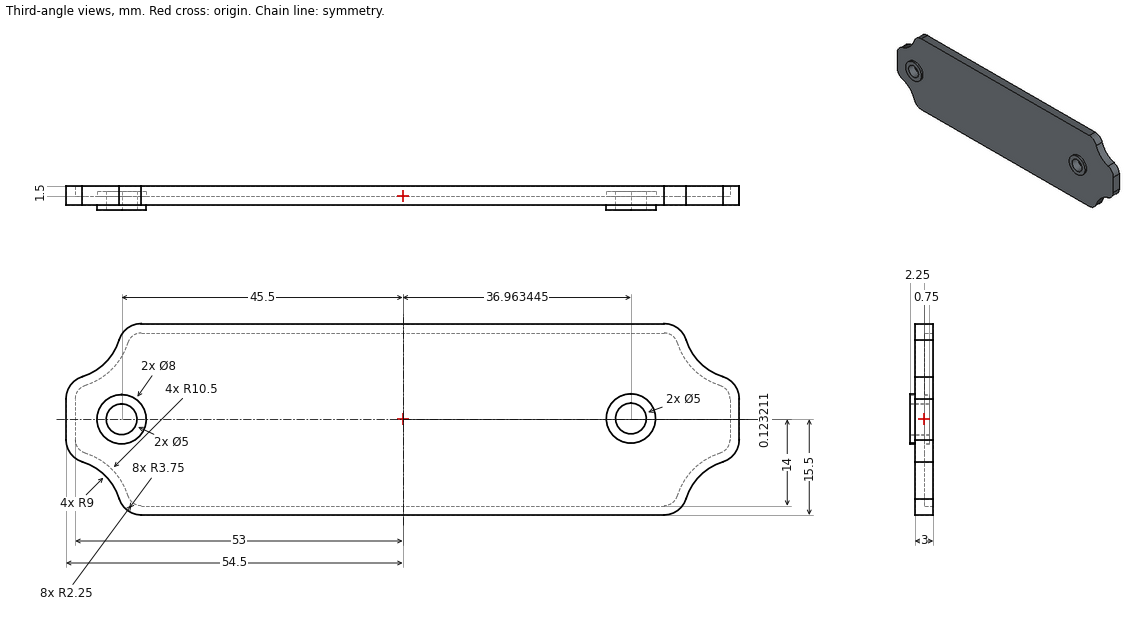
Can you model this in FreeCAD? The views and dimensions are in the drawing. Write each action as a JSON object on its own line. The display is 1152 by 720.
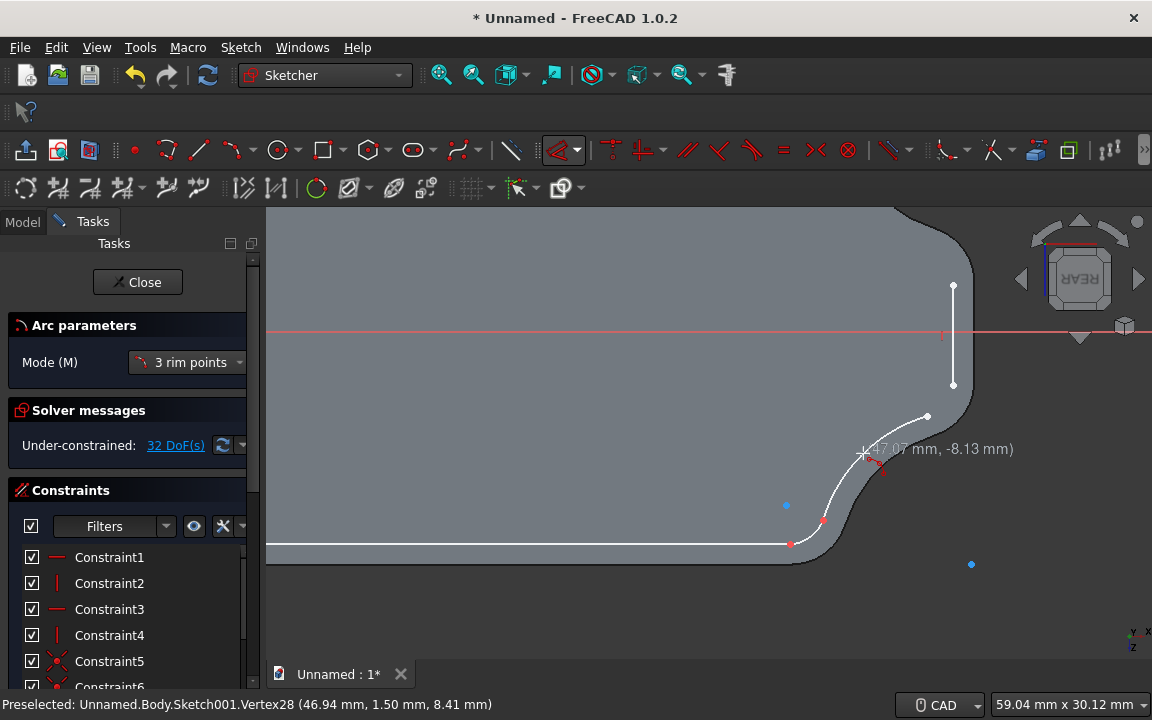
{"action": "left_click", "coordinate": [927, 416]}
{"action": "left_click", "coordinate": [953, 385]}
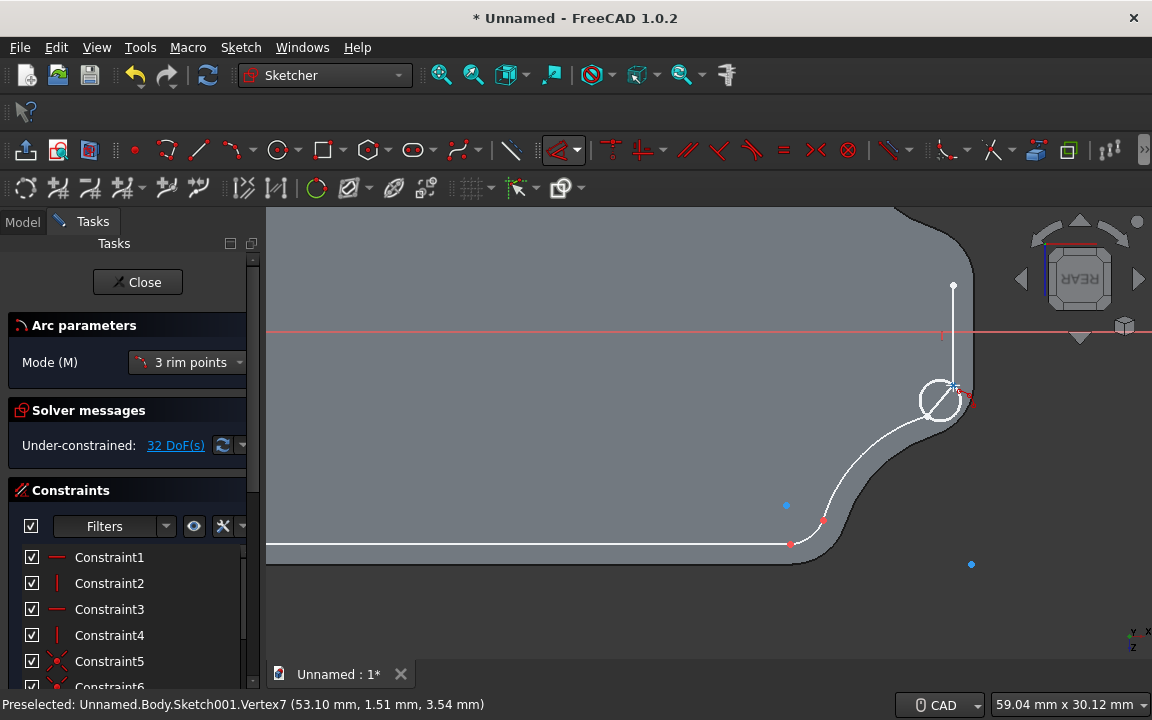
{"action": "scroll", "coordinate": [945, 402], "scroll_direction": "up", "scroll_amount": 5}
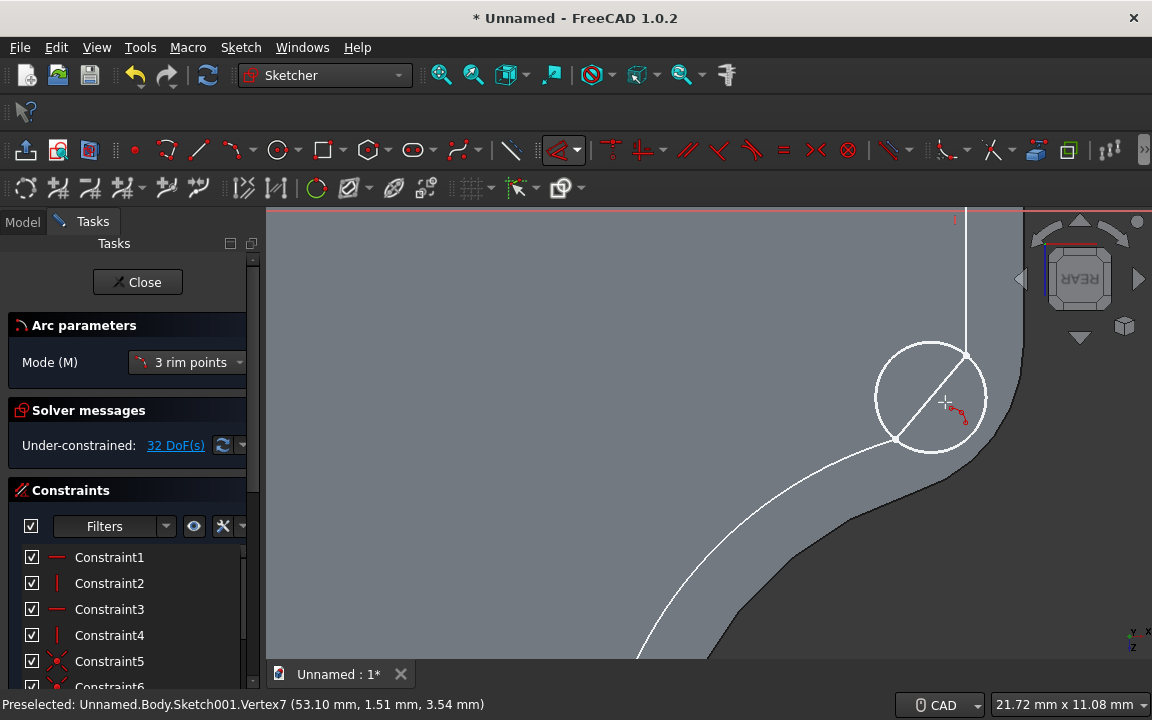
{"action": "left_click", "coordinate": [945, 401]}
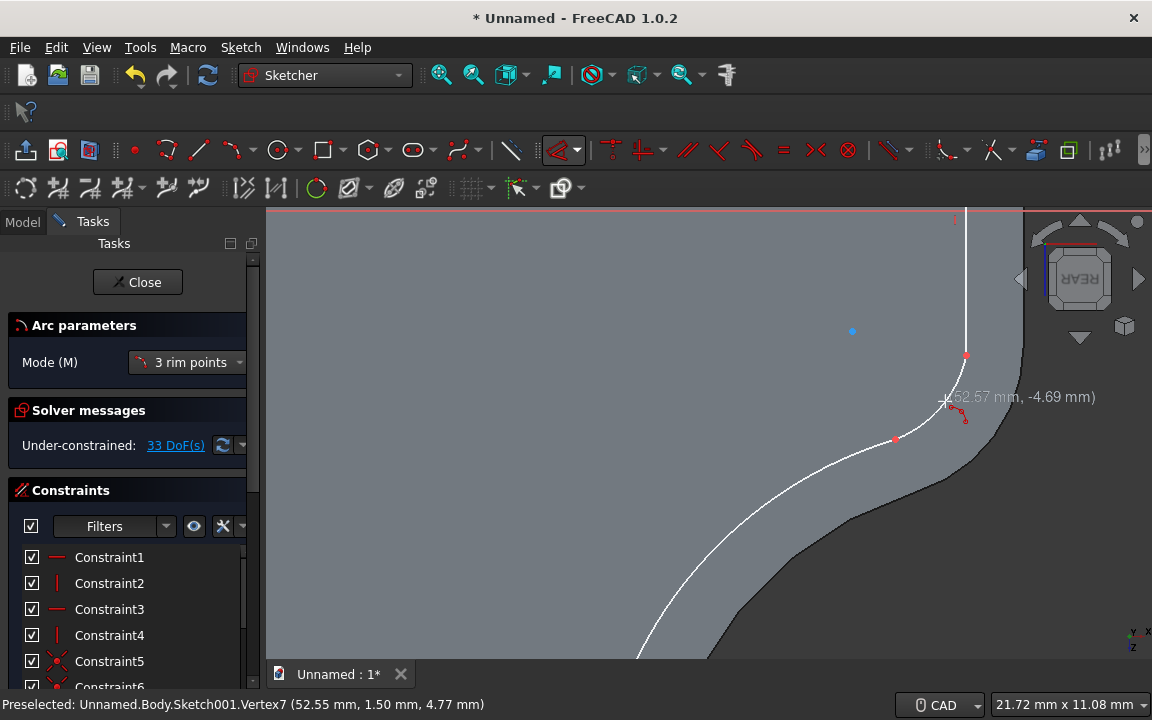
{"action": "scroll", "coordinate": [870, 461], "scroll_direction": "down", "scroll_amount": 11}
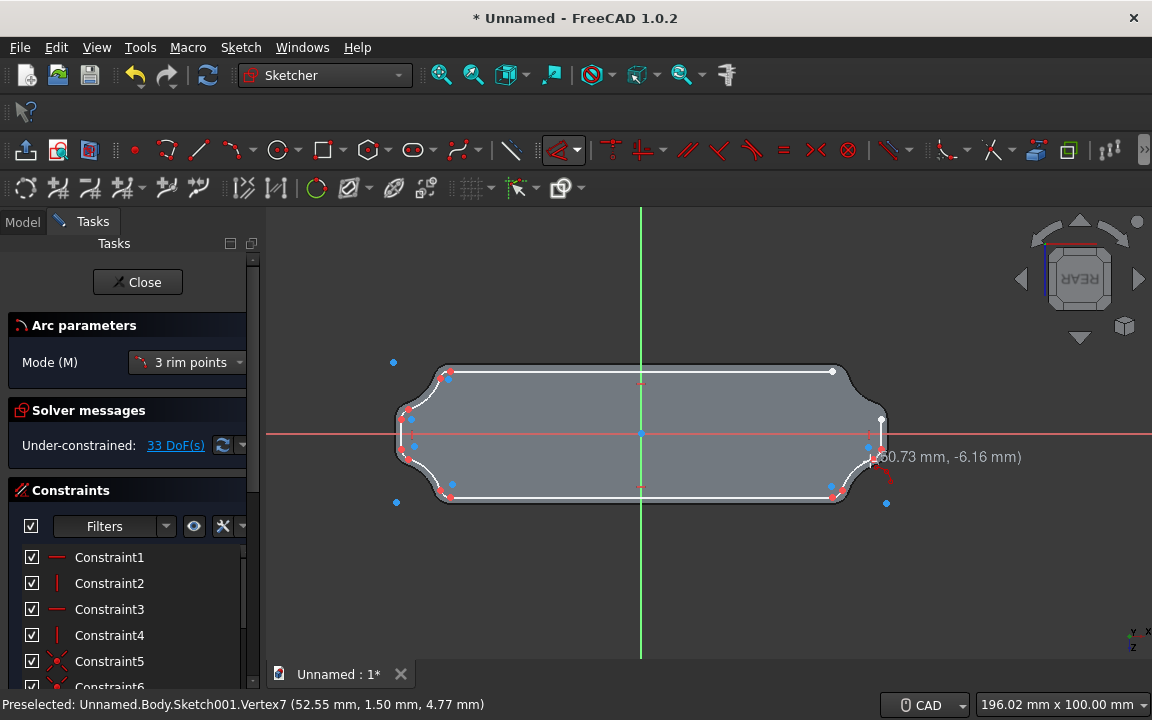
{"action": "left_click", "coordinate": [881, 420]}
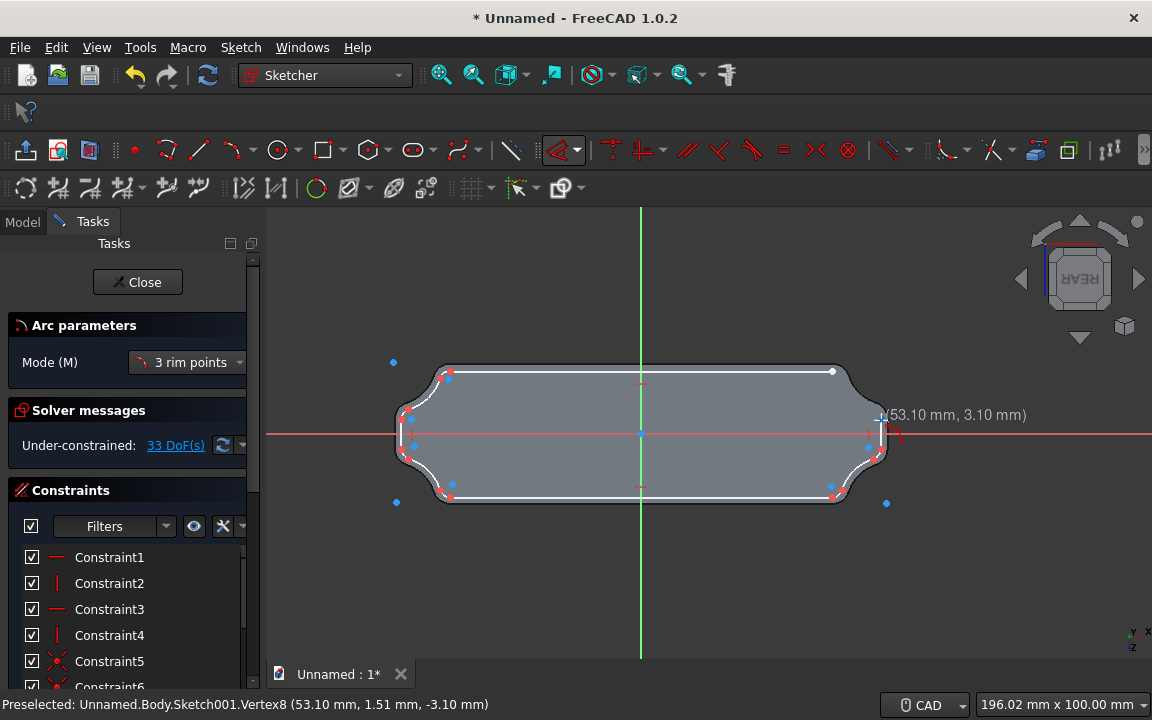
{"action": "scroll", "coordinate": [874, 409], "scroll_direction": "up", "scroll_amount": 2}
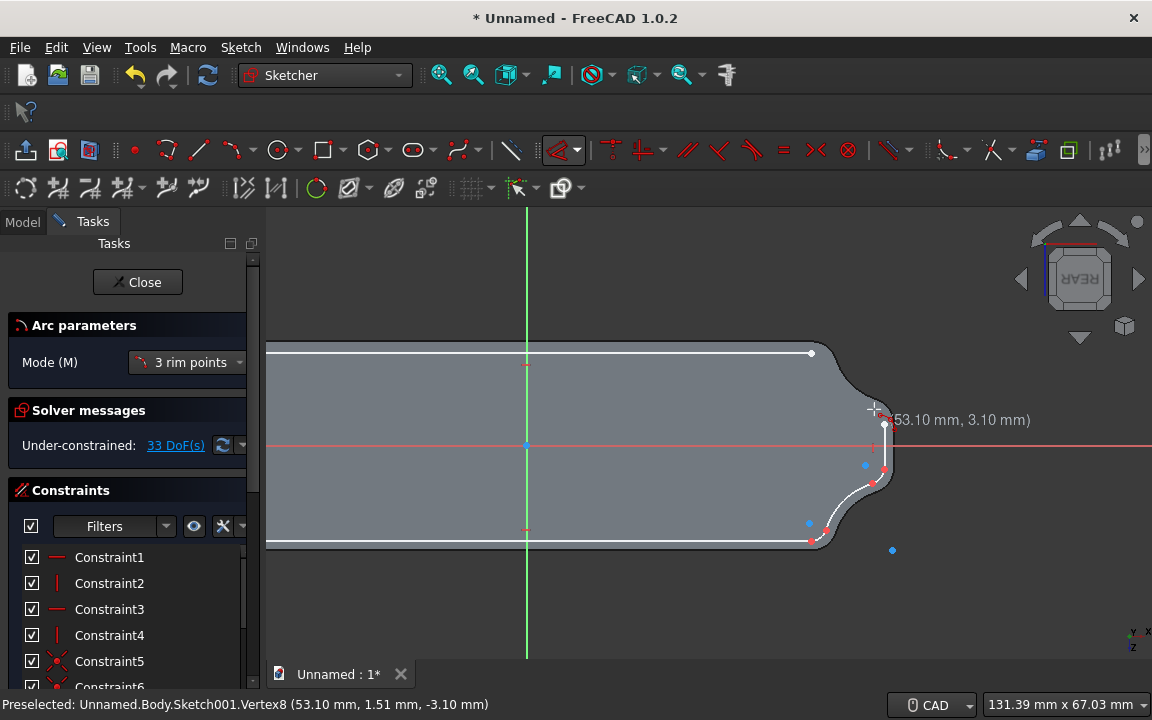
{"action": "left_click", "coordinate": [873, 409]}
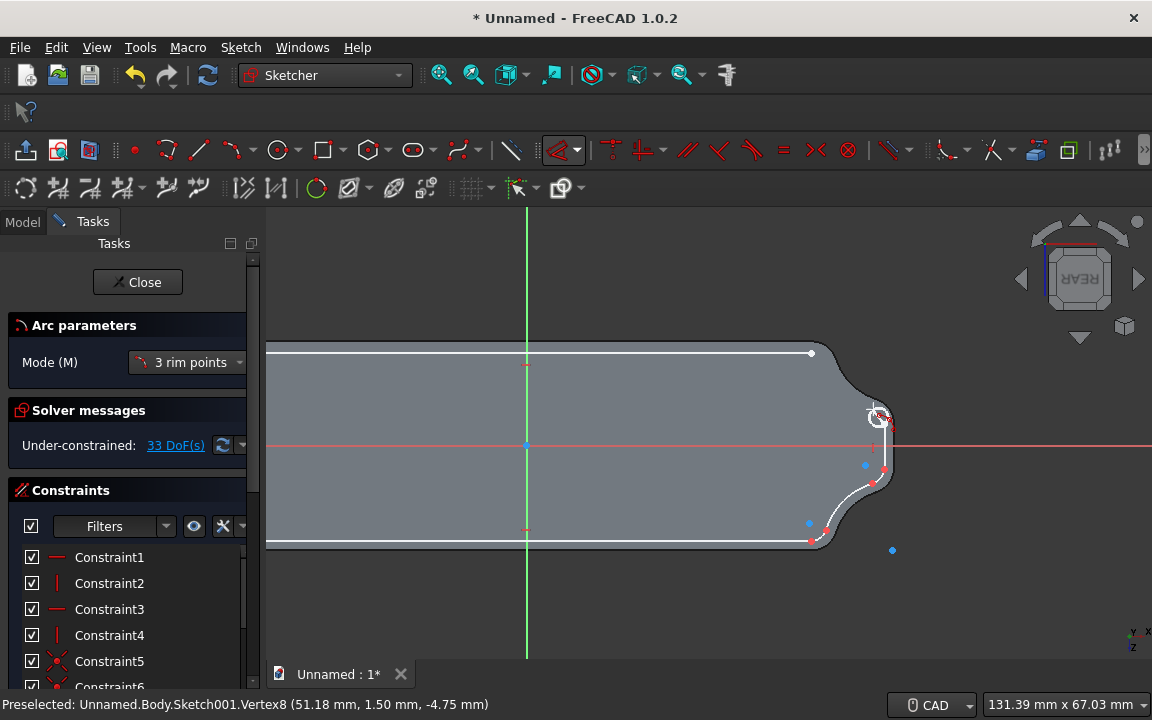
{"action": "scroll", "coordinate": [881, 414], "scroll_direction": "up", "scroll_amount": 9}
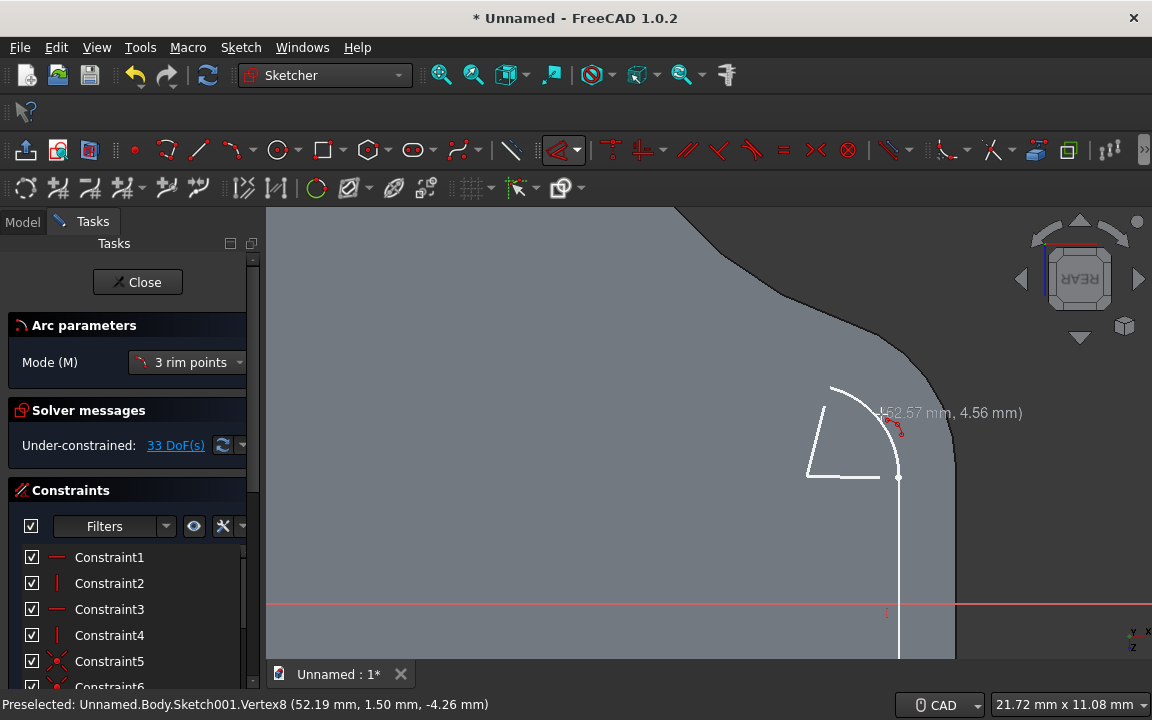
{"action": "left_click", "coordinate": [877, 414]}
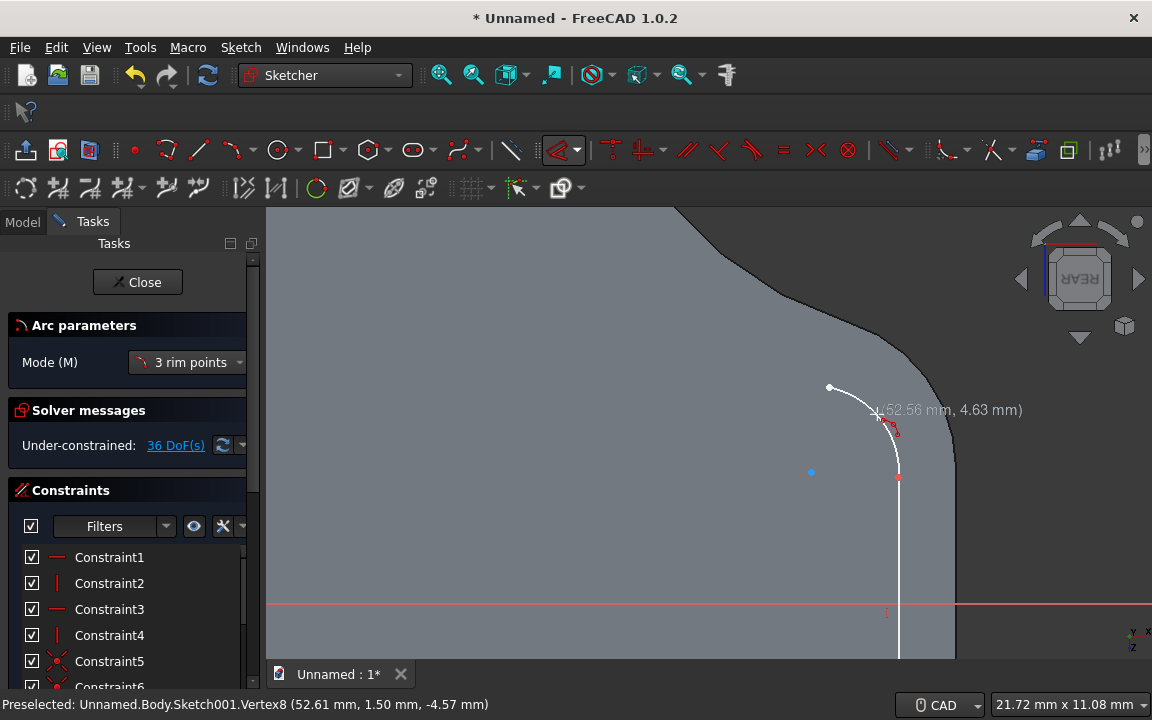
{"action": "scroll", "coordinate": [878, 412], "scroll_direction": "down", "scroll_amount": 11}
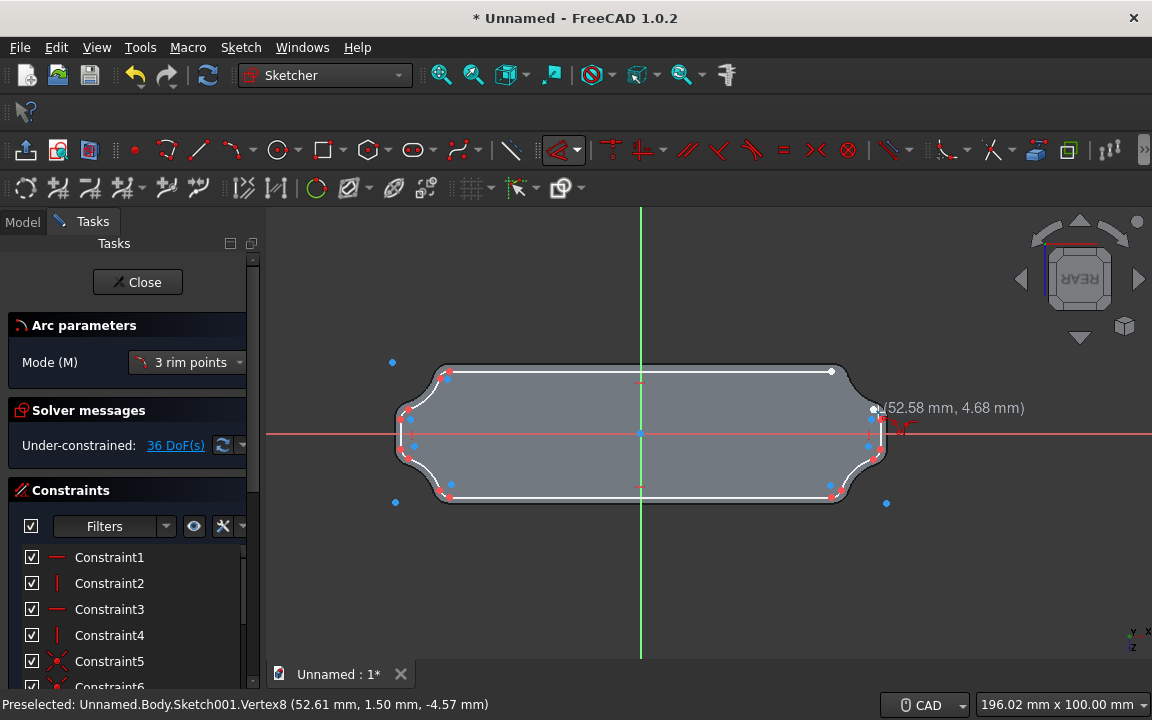
{"action": "scroll", "coordinate": [873, 409], "scroll_direction": "up", "scroll_amount": 3}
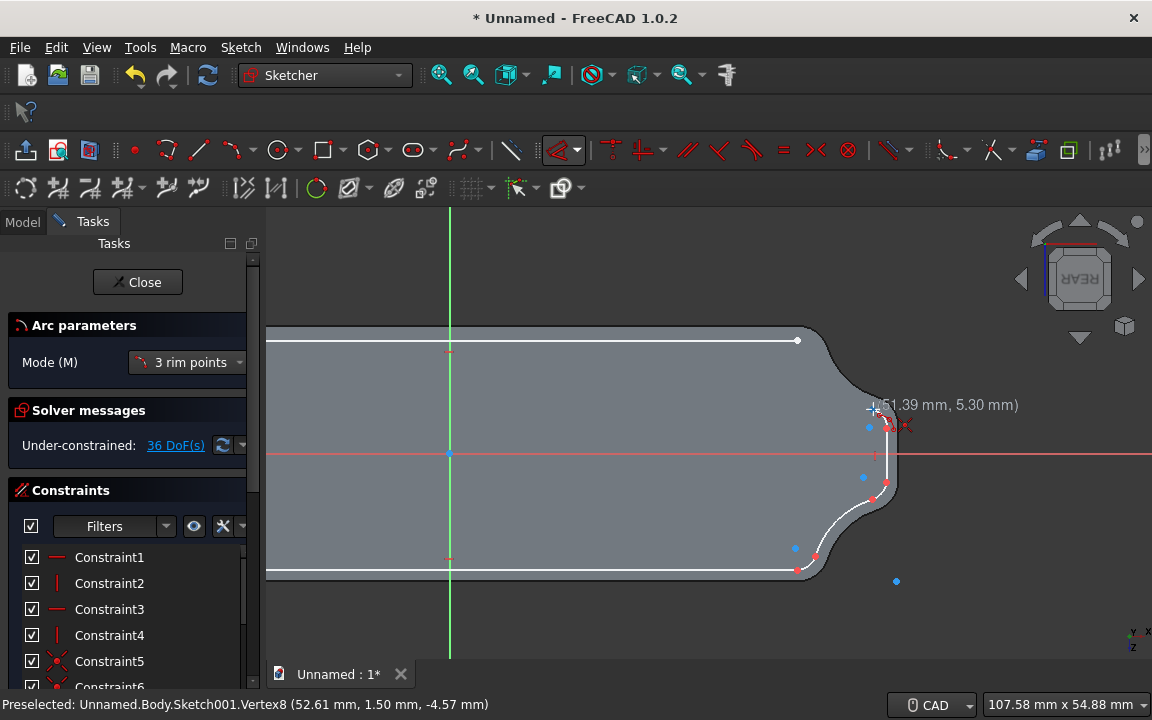
{"action": "left_click", "coordinate": [873, 410]}
{"action": "left_click", "coordinate": [816, 351]}